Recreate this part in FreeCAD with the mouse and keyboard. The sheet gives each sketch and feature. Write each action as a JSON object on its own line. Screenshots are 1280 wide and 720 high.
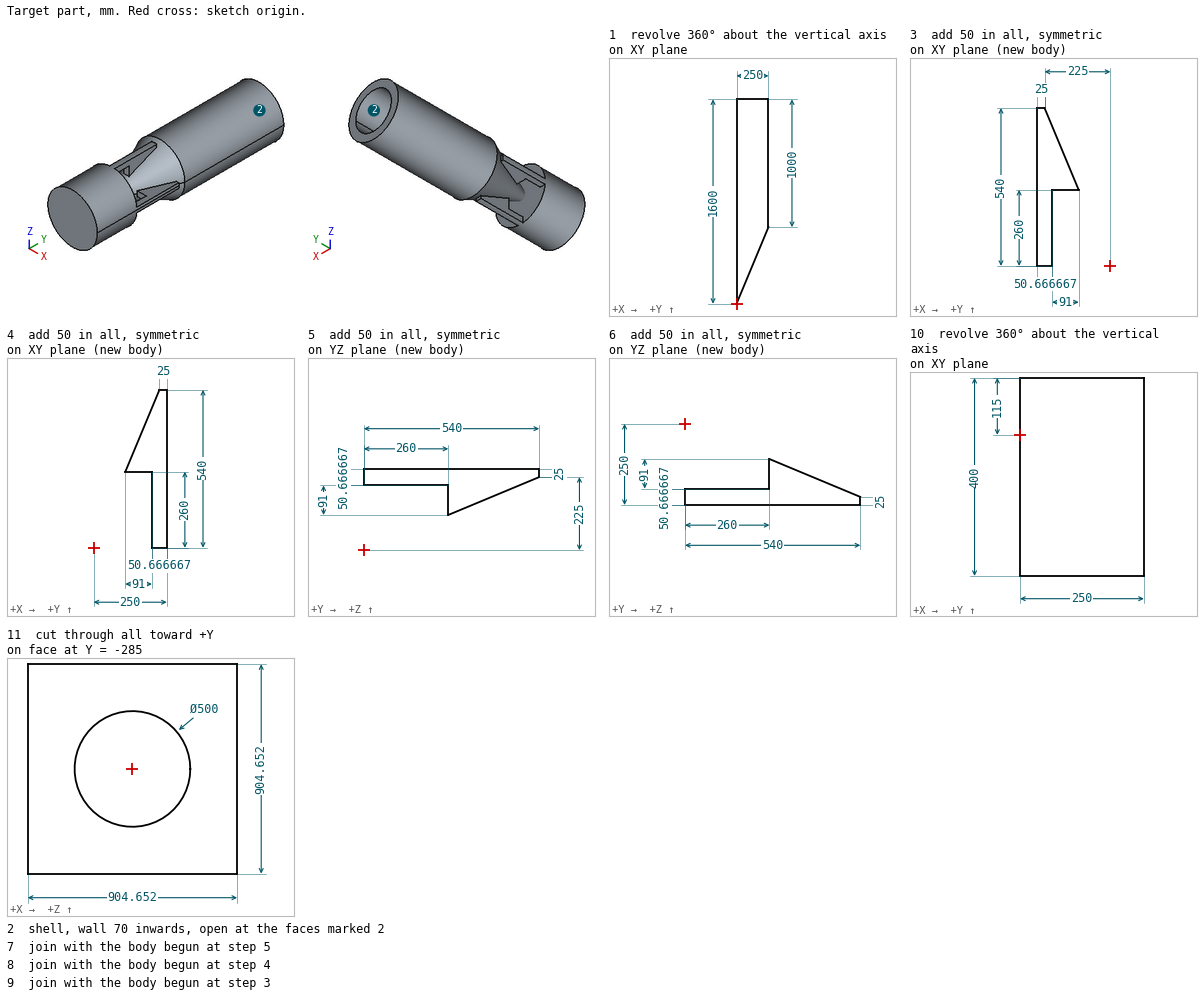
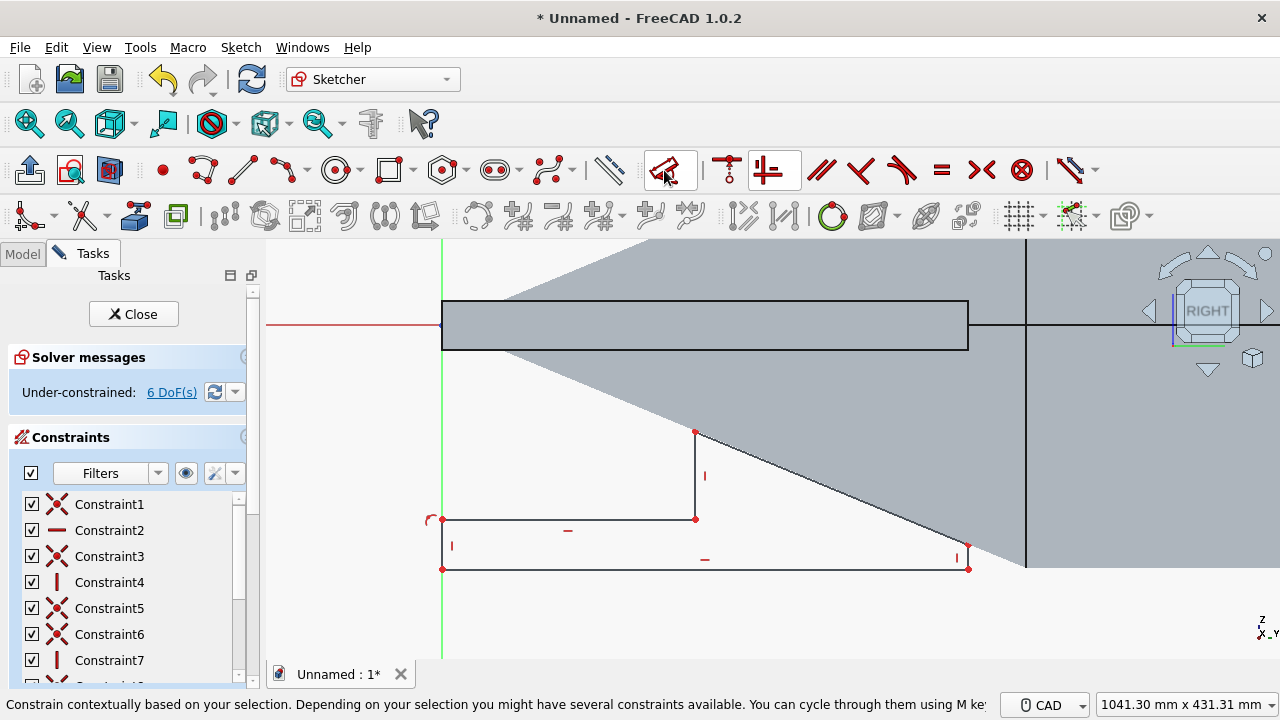
{"action": "scroll", "coordinate": [968, 560], "scroll_direction": "up", "scroll_amount": 3}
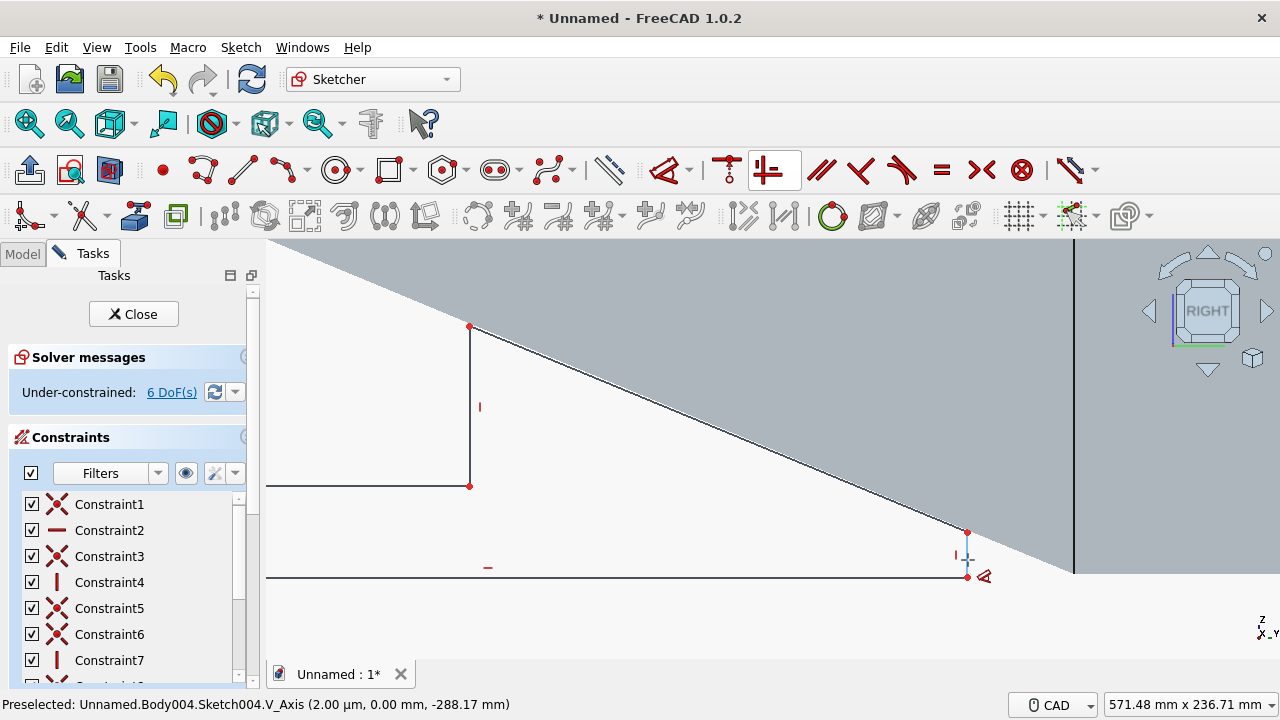
{"action": "left_click", "coordinate": [967, 559]}
{"action": "left_click", "coordinate": [1001, 555]}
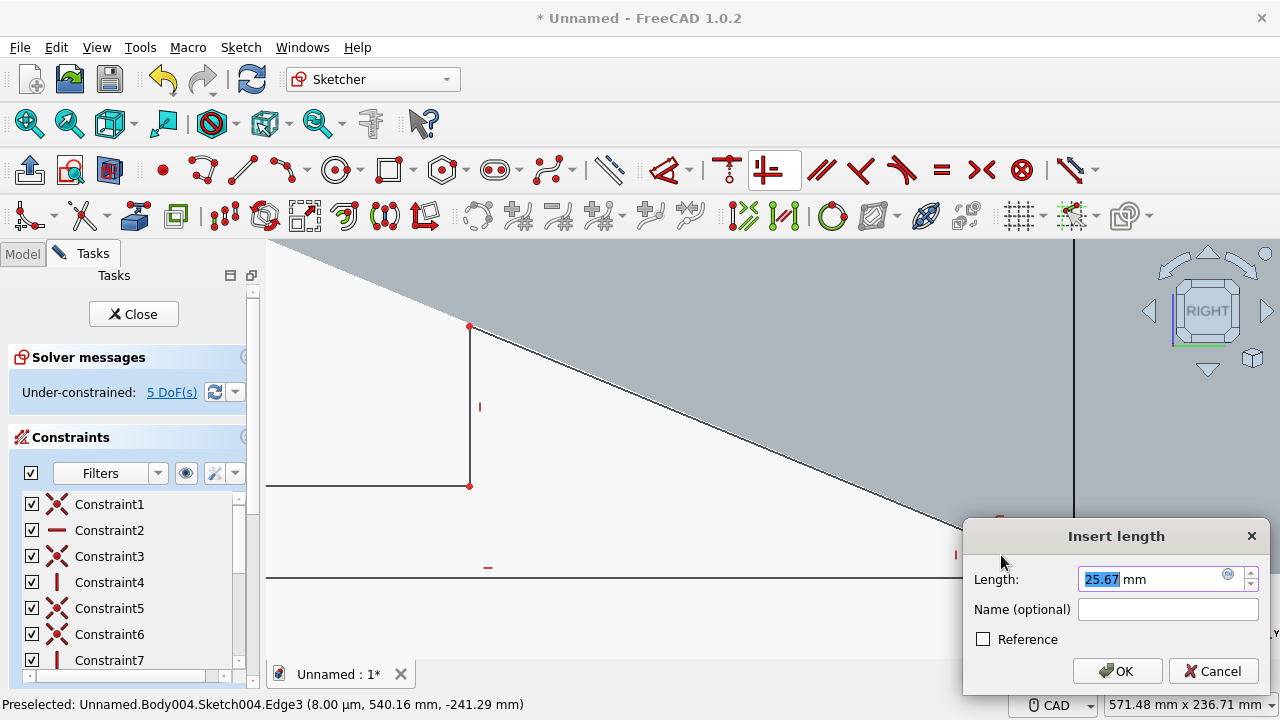
{"action": "type", "text": "25"}
{"action": "key", "text": "Return"}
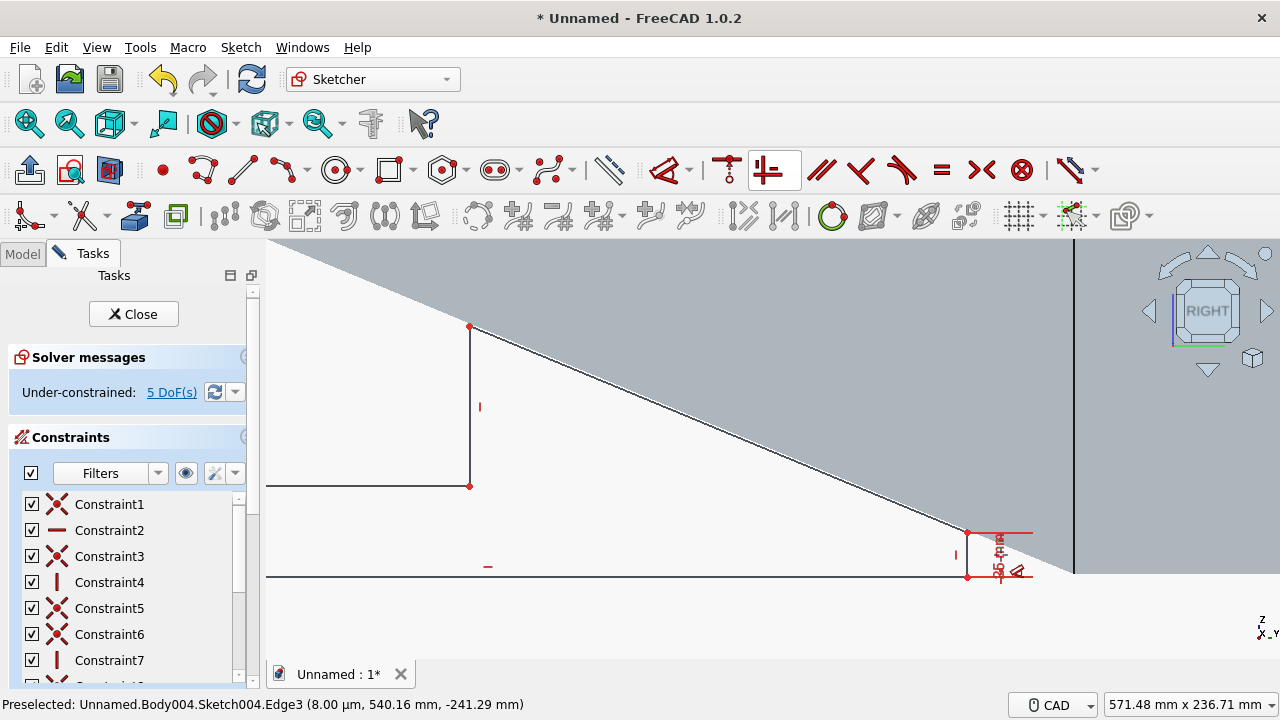
{"action": "left_click", "coordinate": [470, 374]}
{"action": "left_click", "coordinate": [436, 406]}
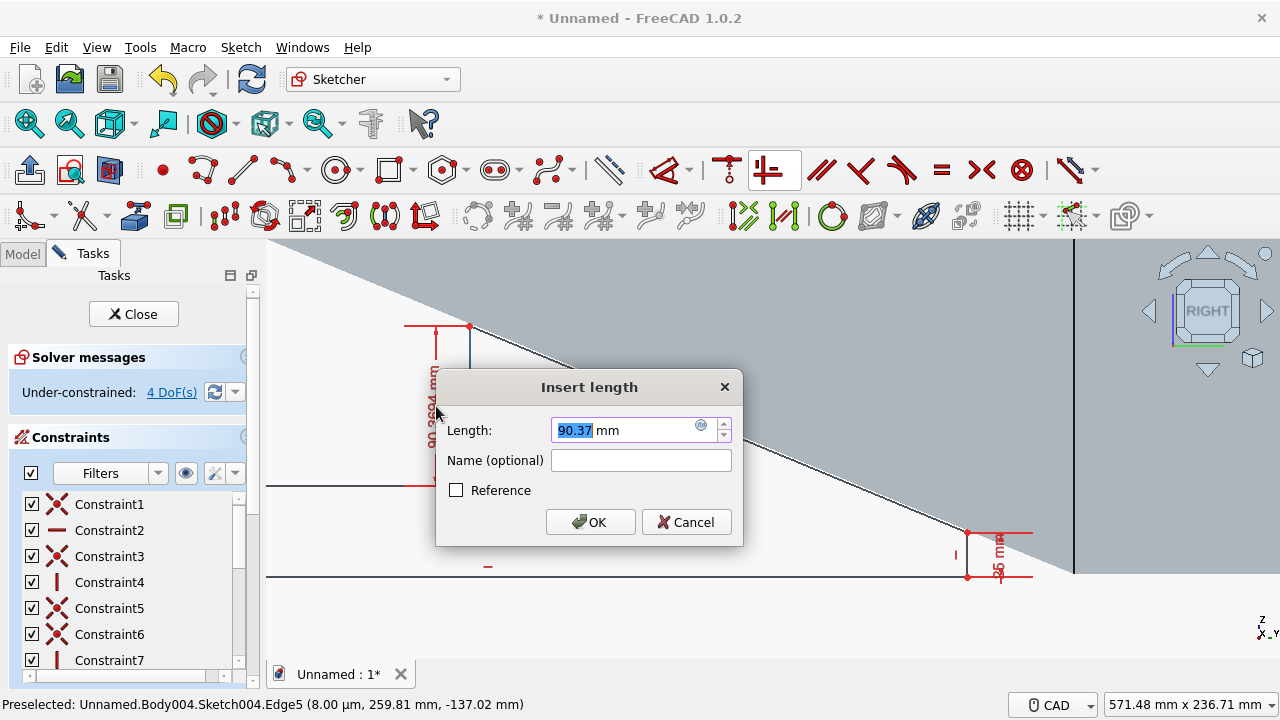
{"action": "type", "text": "91"}
{"action": "key", "text": "Return"}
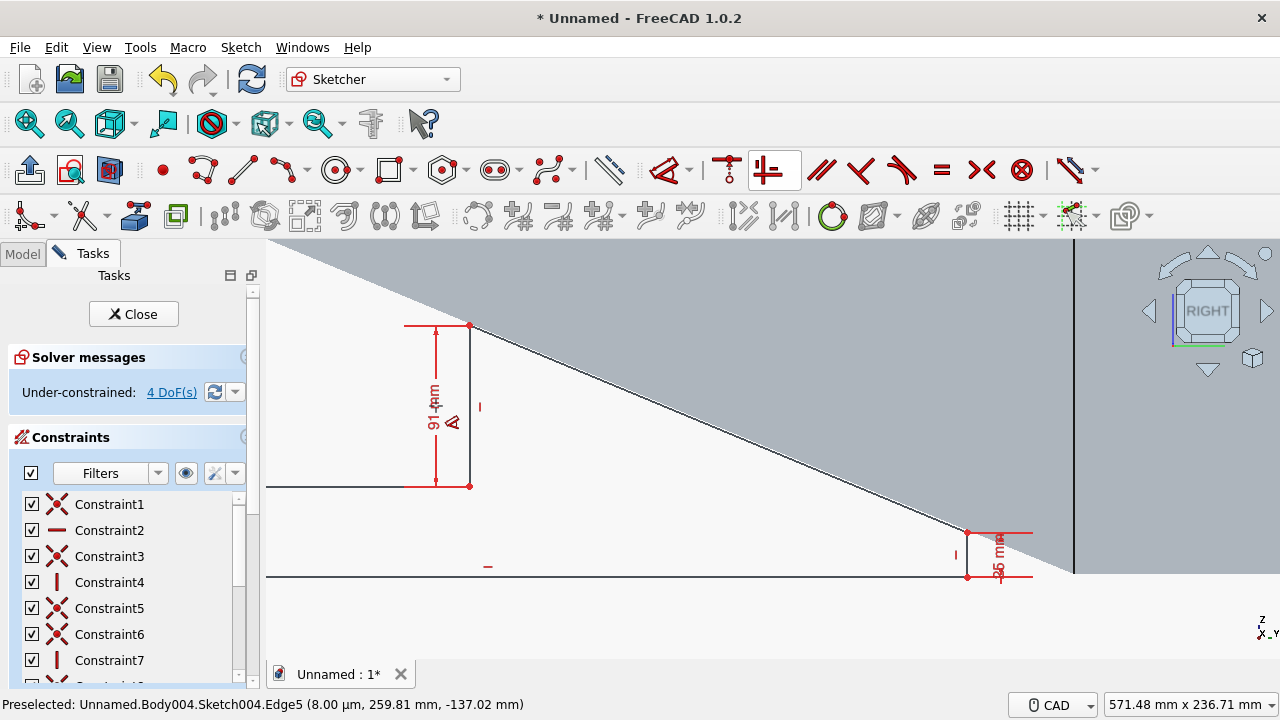
{"action": "left_click", "coordinate": [297, 577]}
{"action": "left_click", "coordinate": [631, 611]}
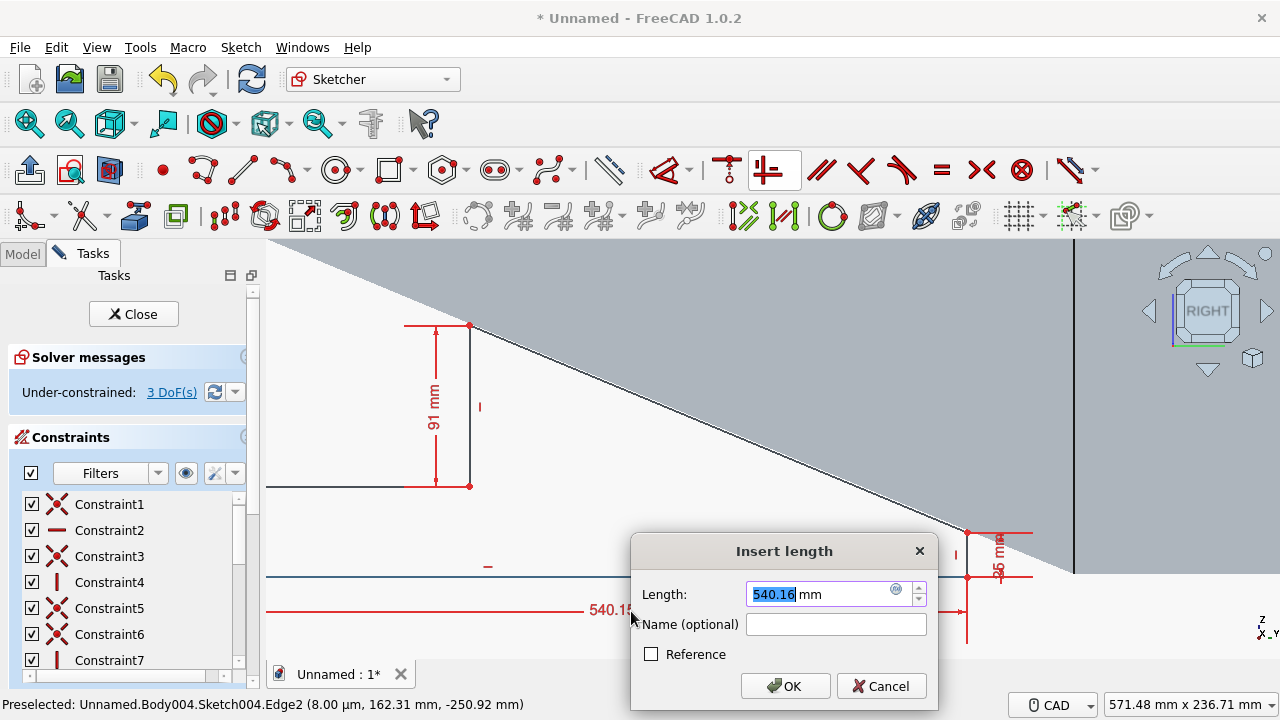
{"action": "type", "text": "540"}
{"action": "key", "text": "Return"}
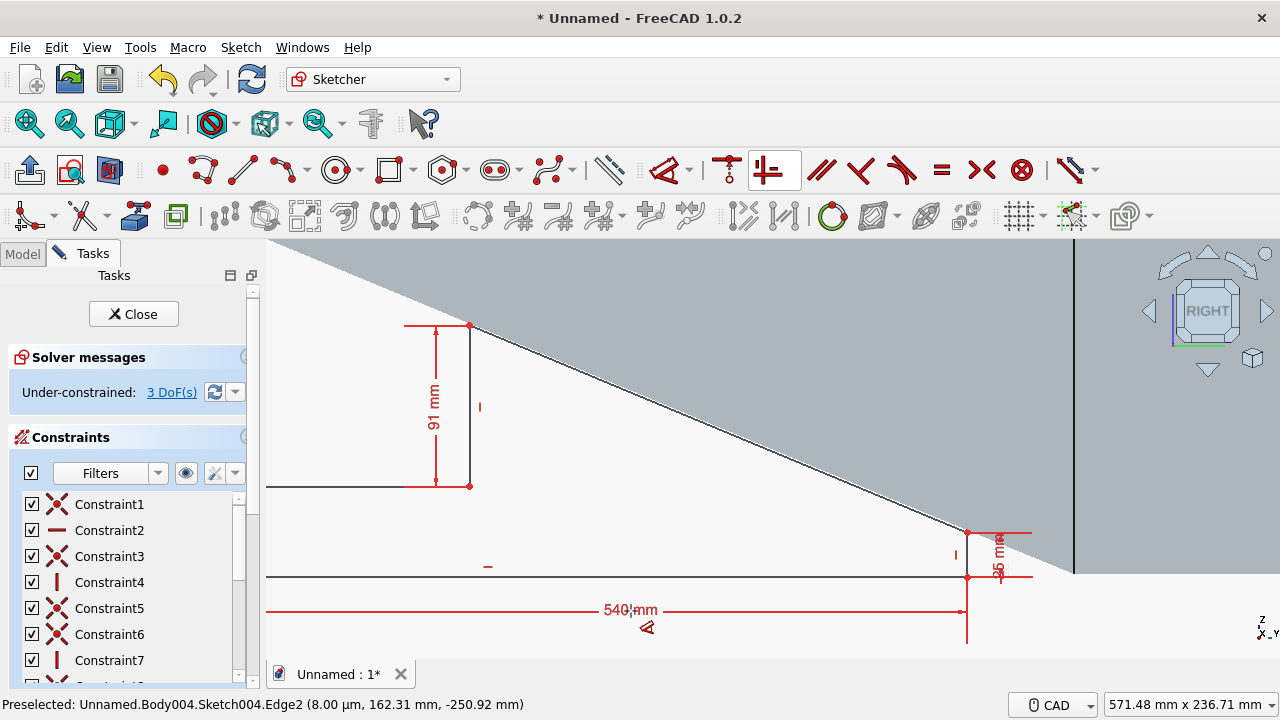
{"action": "left_click", "coordinate": [332, 487]}
{"action": "left_click", "coordinate": [382, 521]}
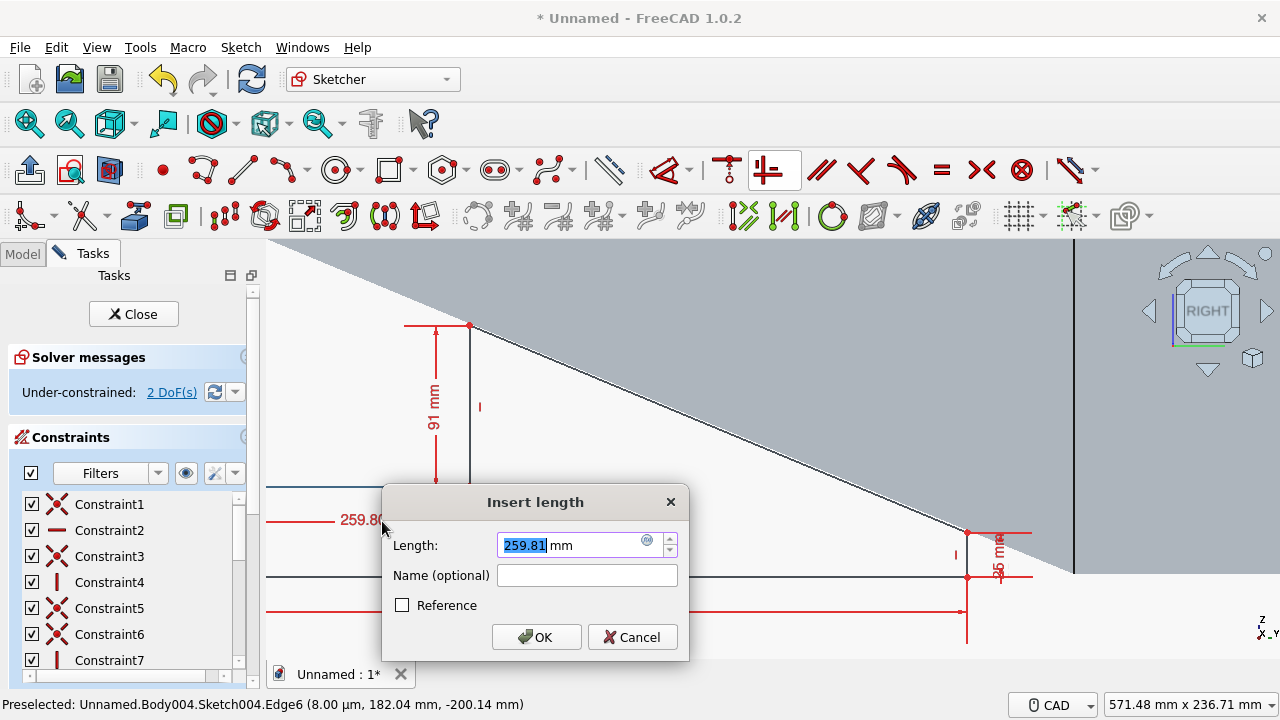
{"action": "type", "text": "260"}
{"action": "key", "text": "Return"}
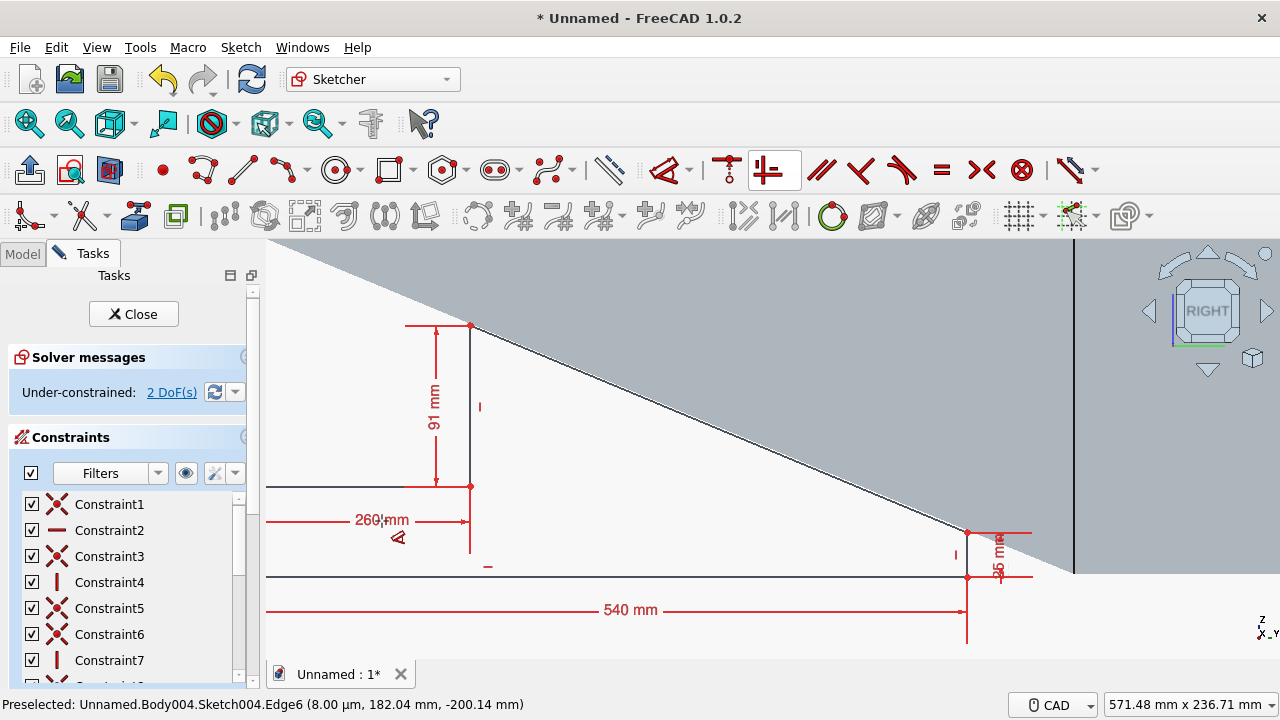
{"action": "scroll", "coordinate": [968, 565], "scroll_direction": "down", "scroll_amount": 3}